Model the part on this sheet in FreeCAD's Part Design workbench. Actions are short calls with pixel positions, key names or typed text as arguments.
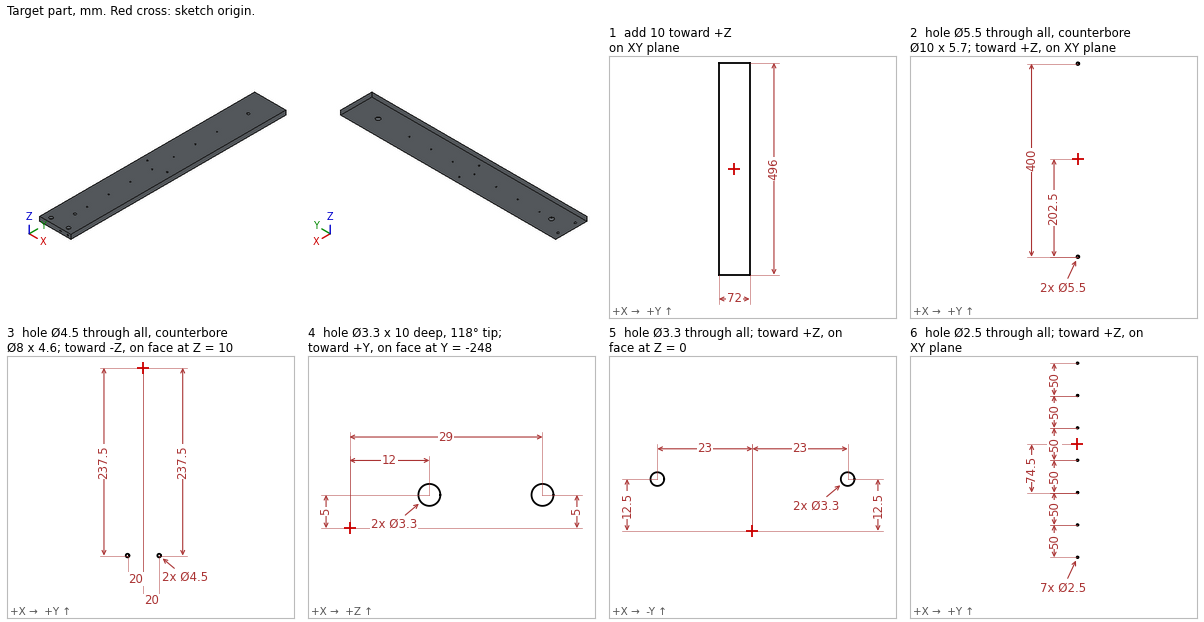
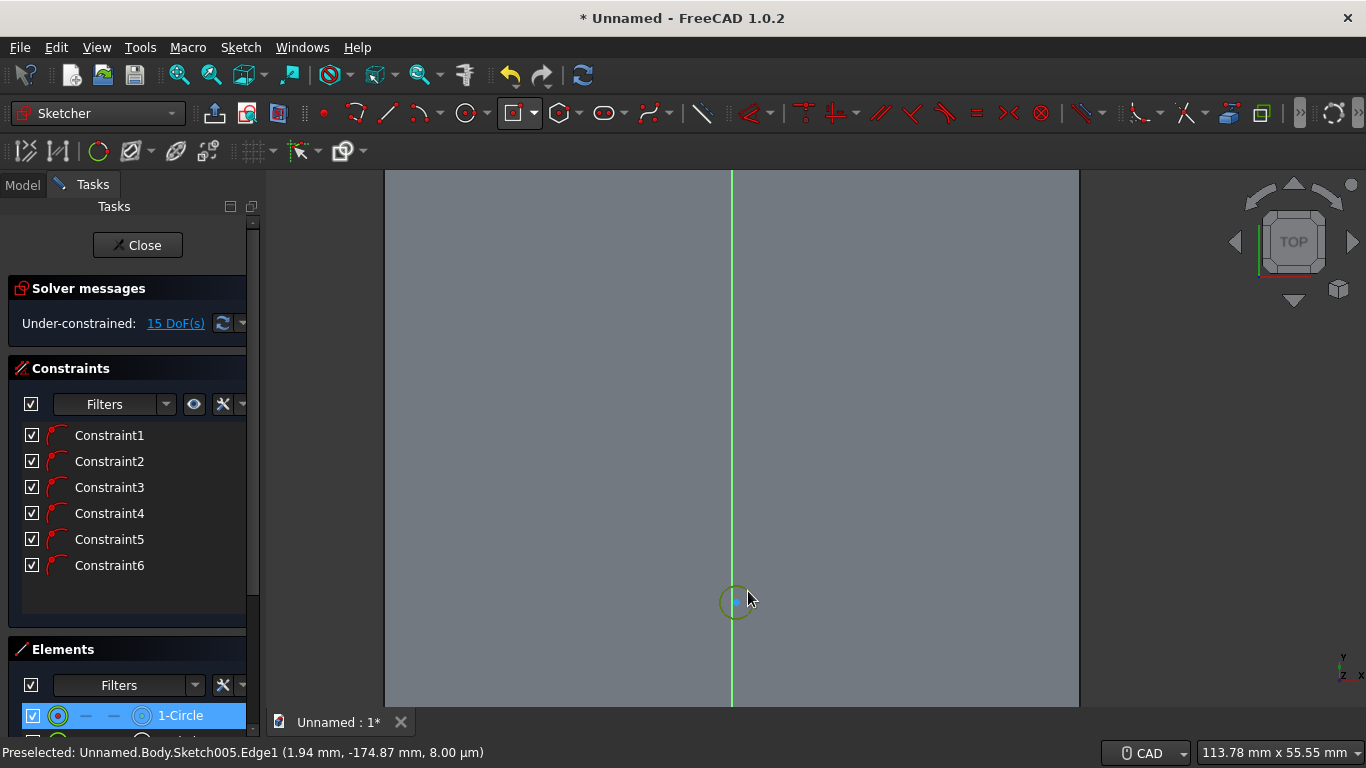
scroll(749, 600, down, 11)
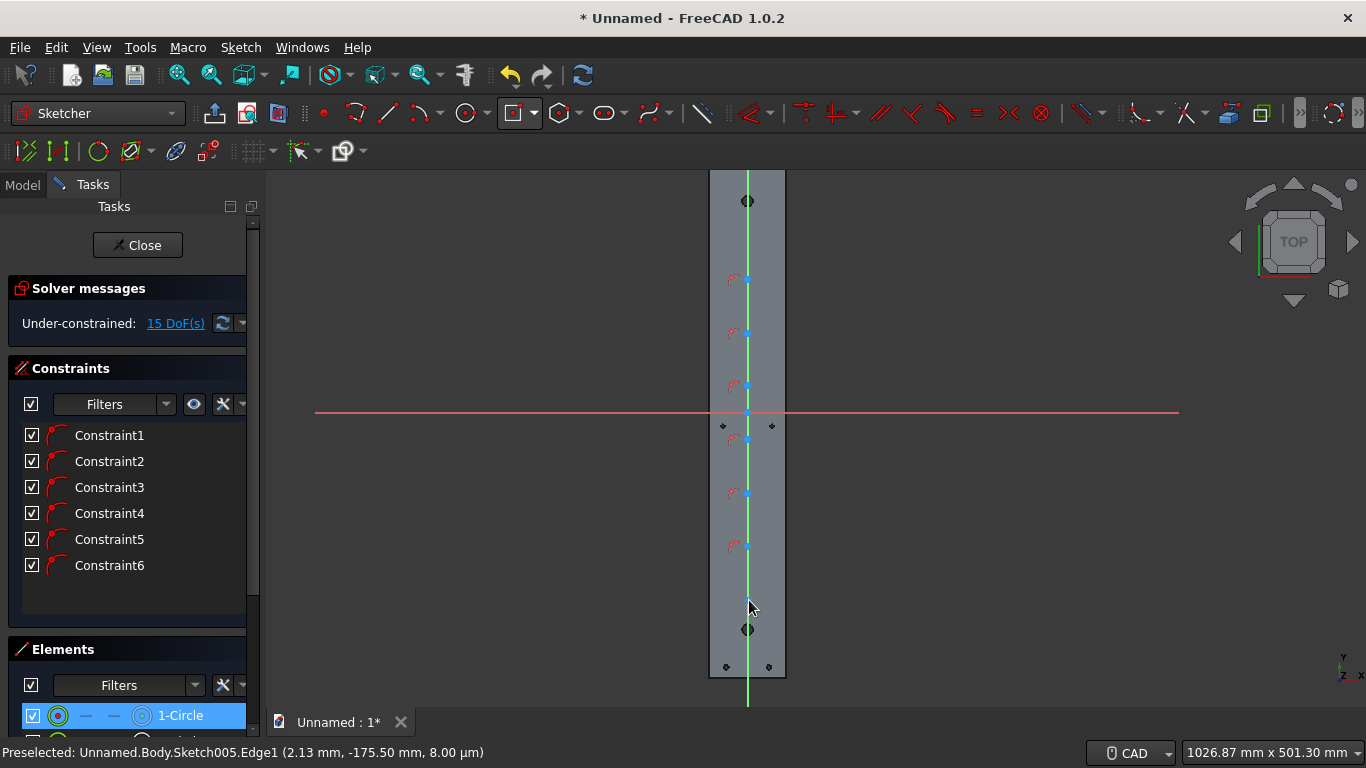
scroll(749, 546, up, 12)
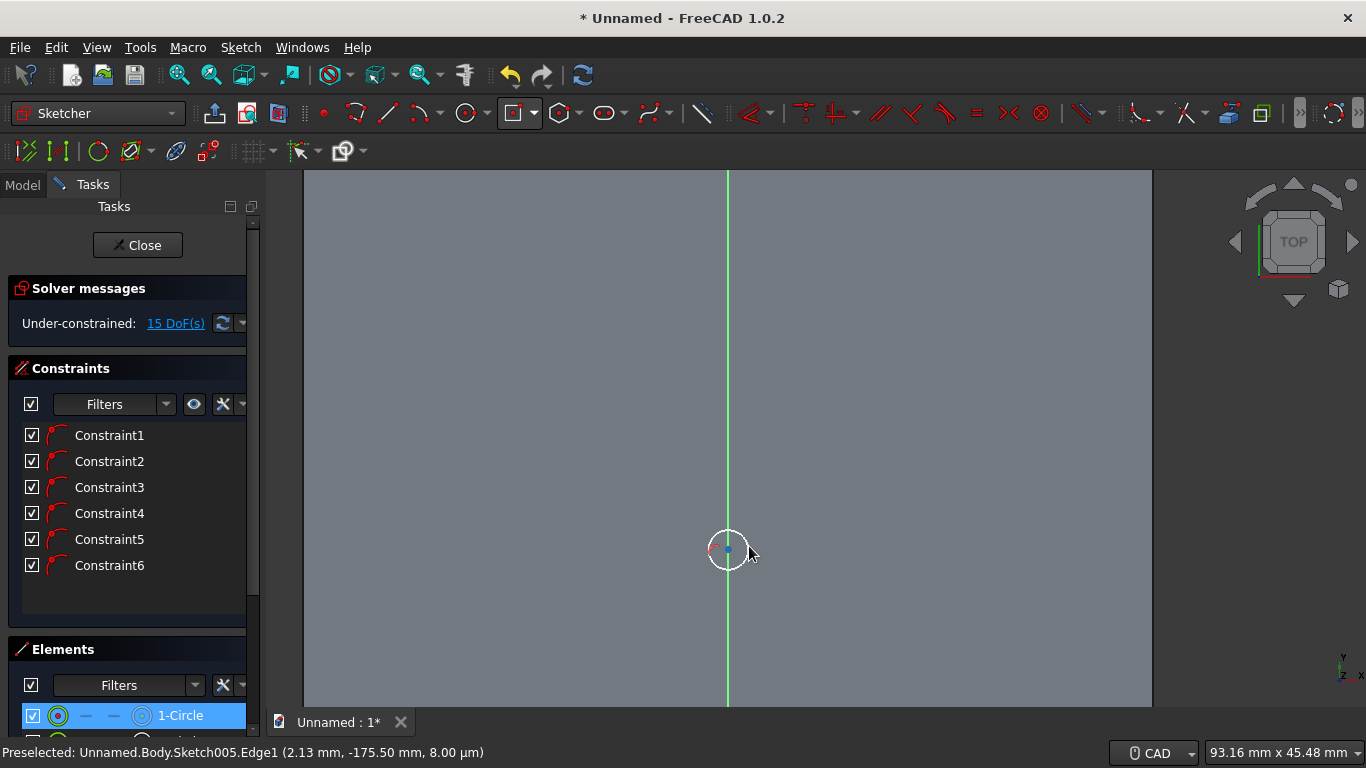
click(742, 536)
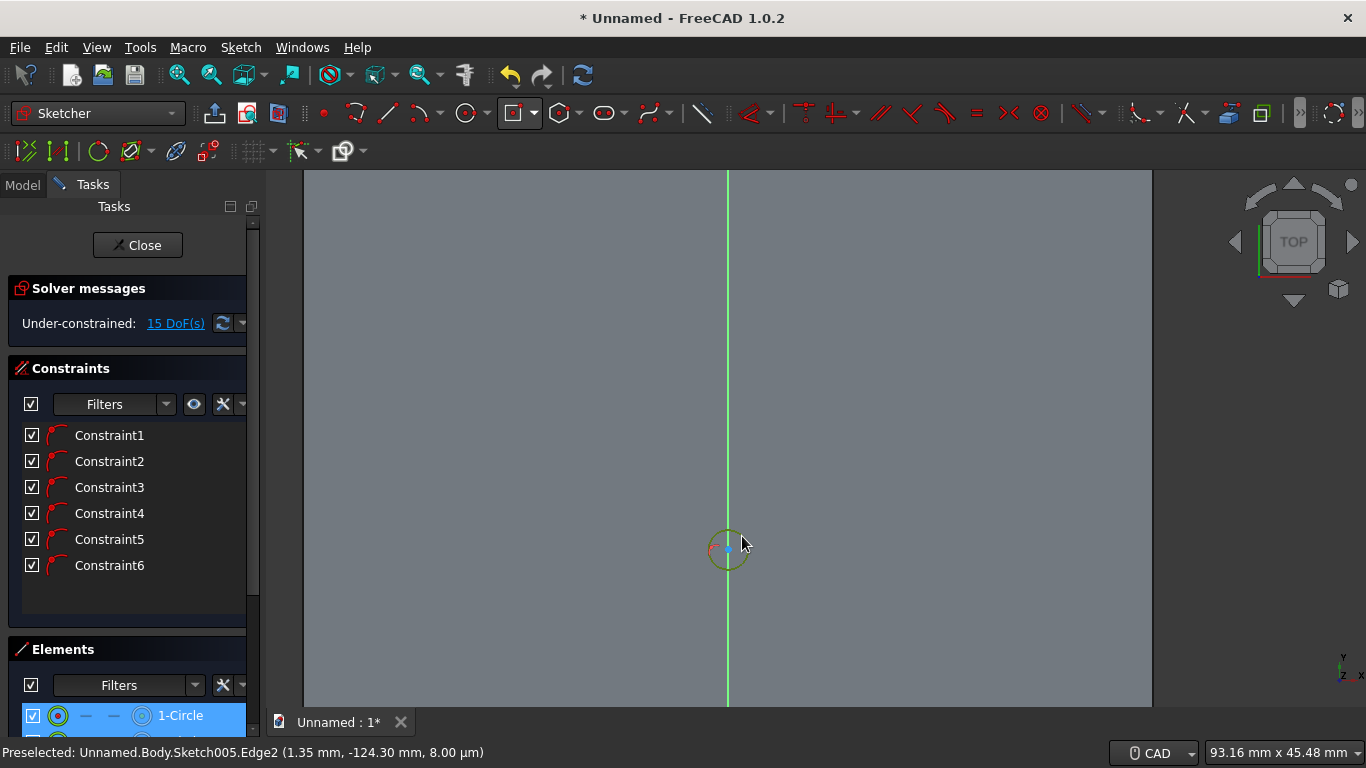
scroll(749, 546, down, 12)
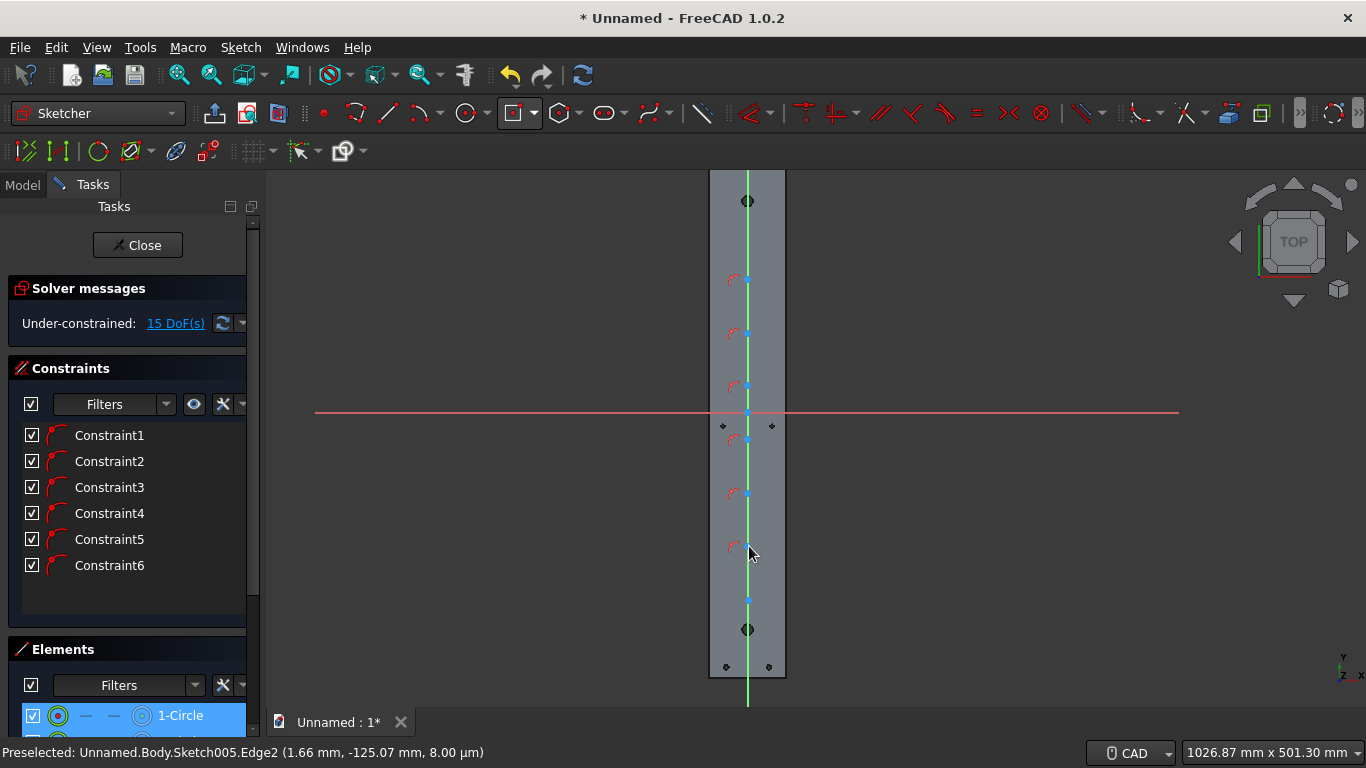
scroll(749, 492, up, 11)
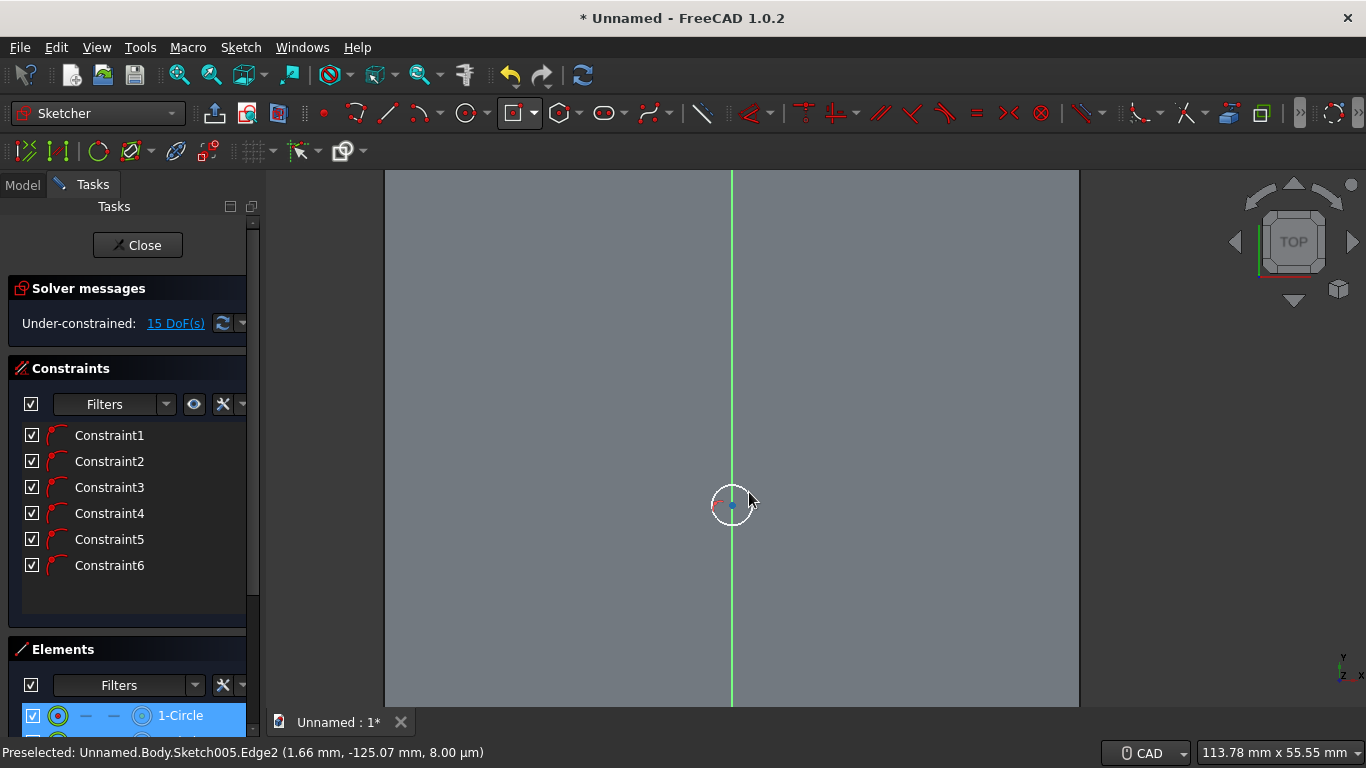
click(746, 491)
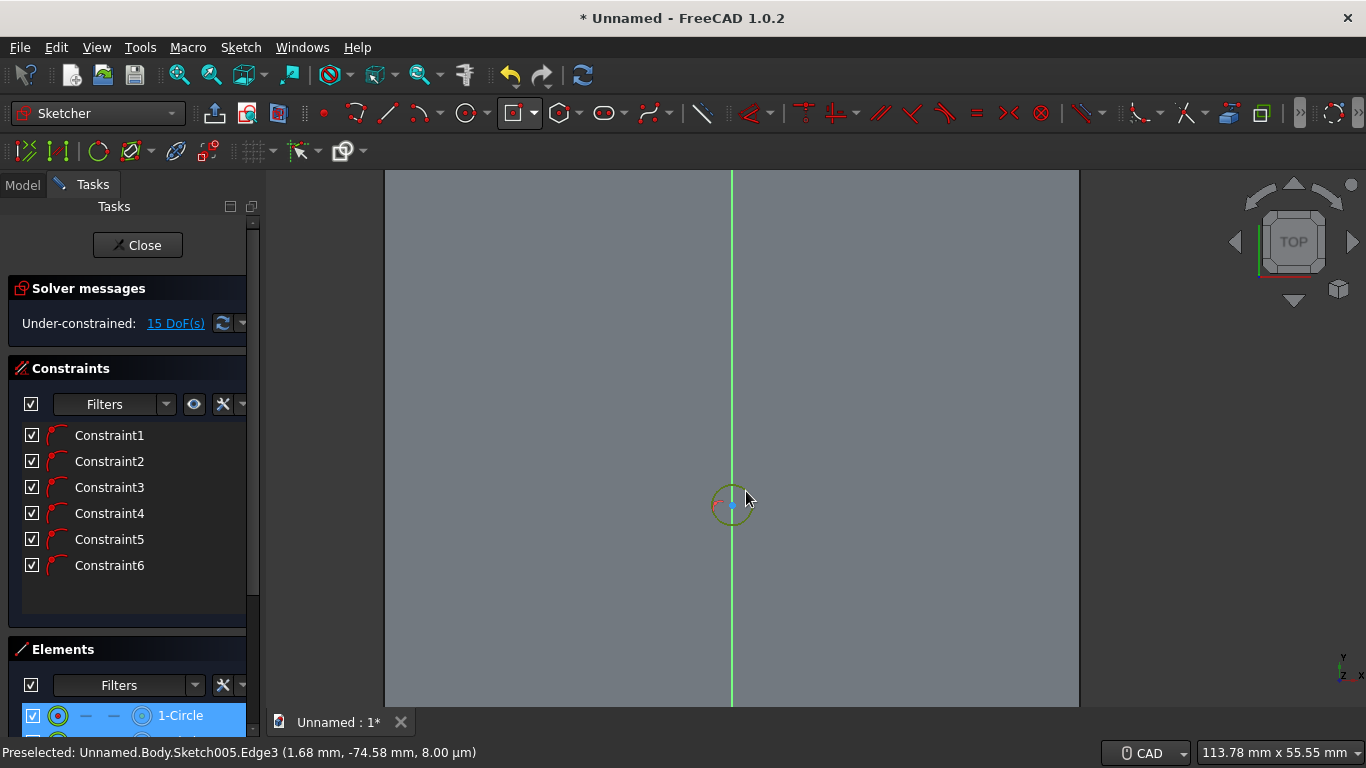
scroll(749, 492, down, 11)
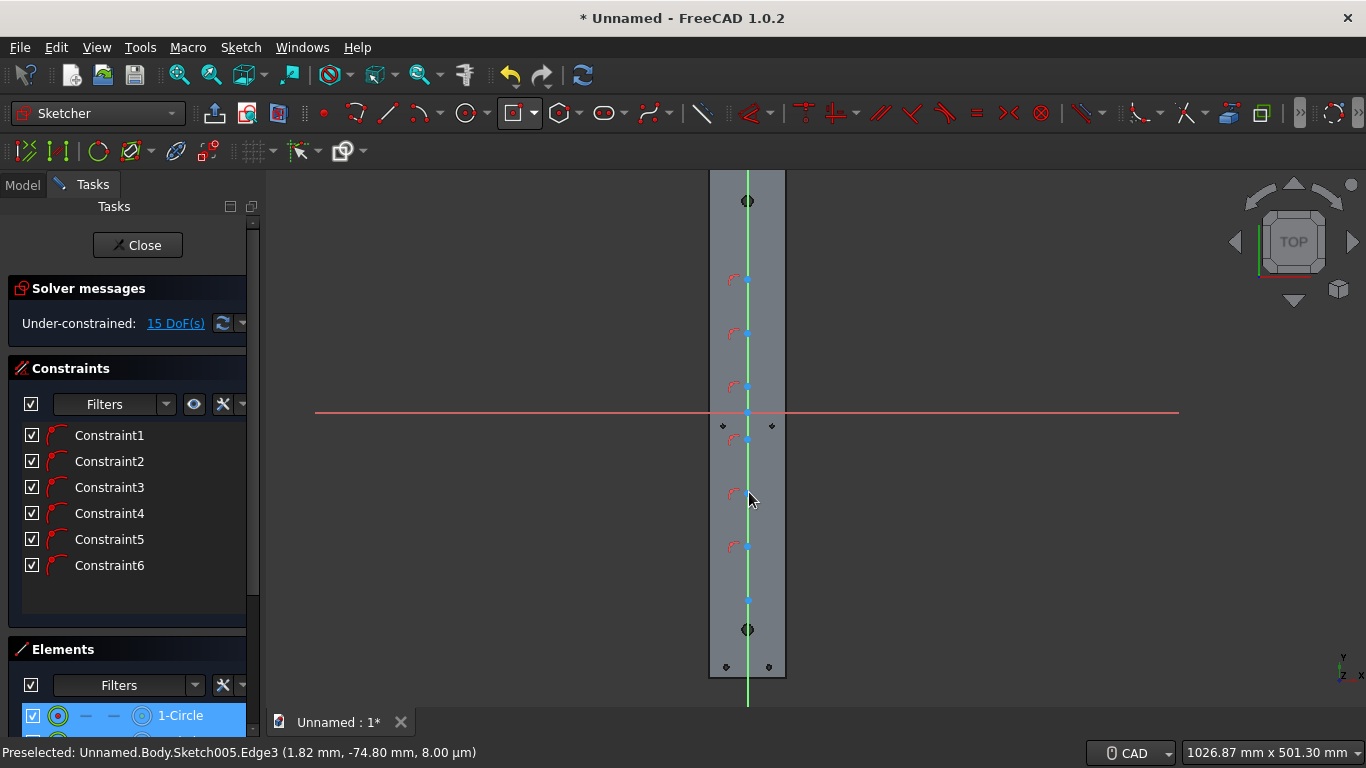
scroll(749, 439, up, 12)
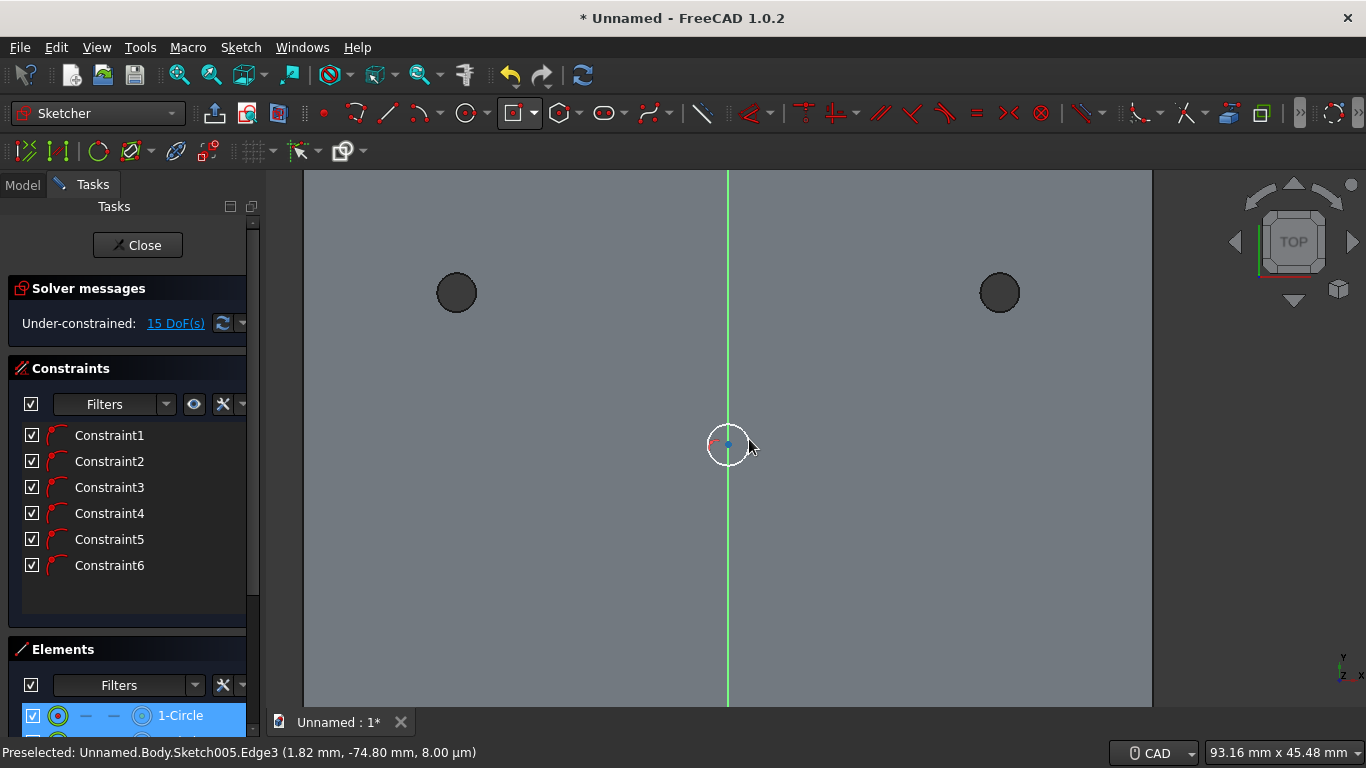
click(743, 430)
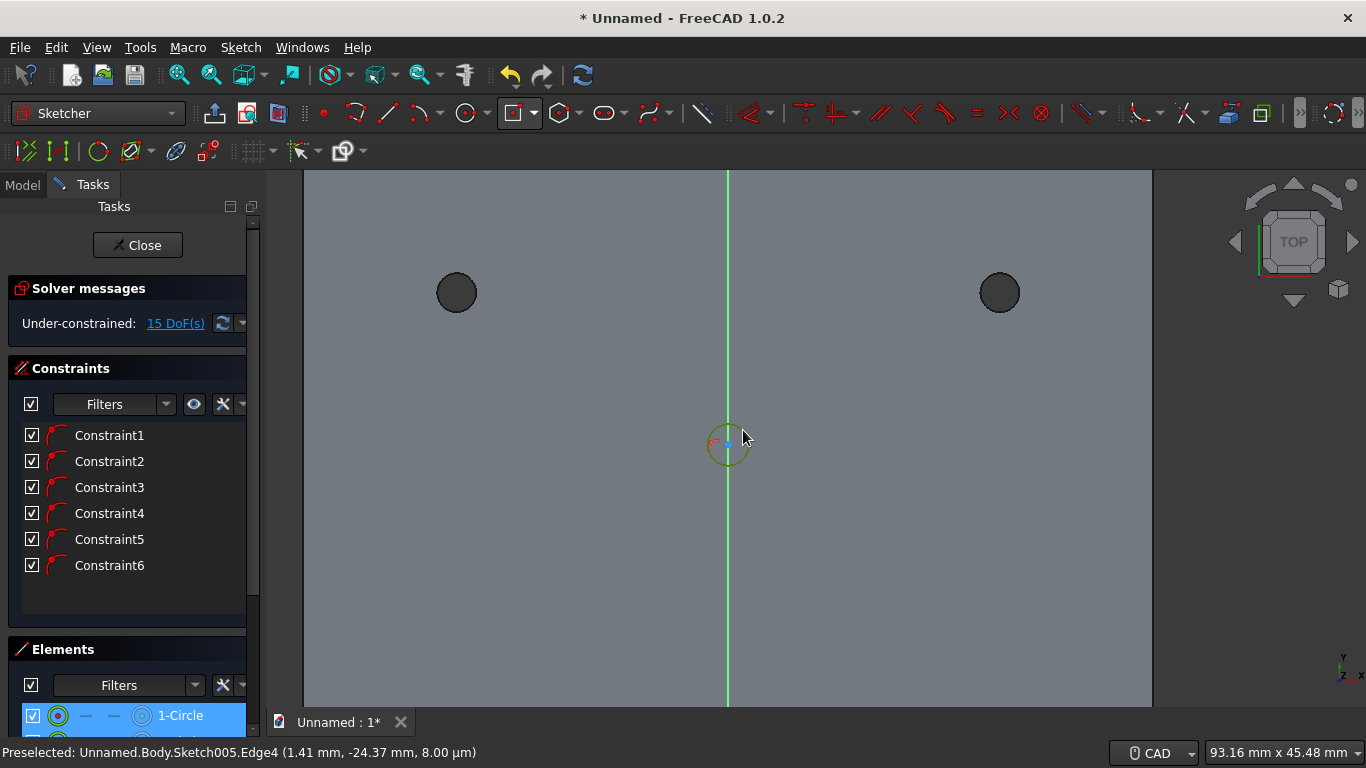
scroll(749, 439, down, 12)